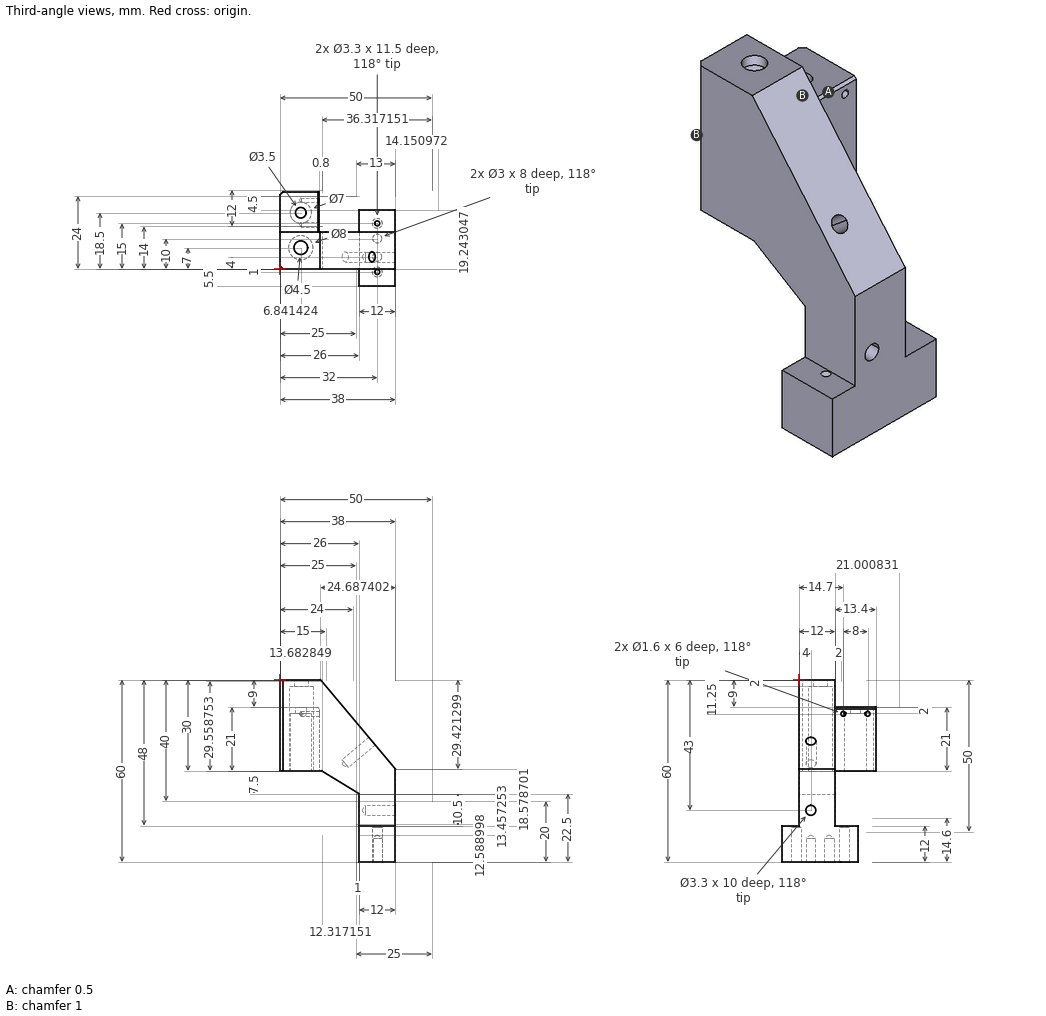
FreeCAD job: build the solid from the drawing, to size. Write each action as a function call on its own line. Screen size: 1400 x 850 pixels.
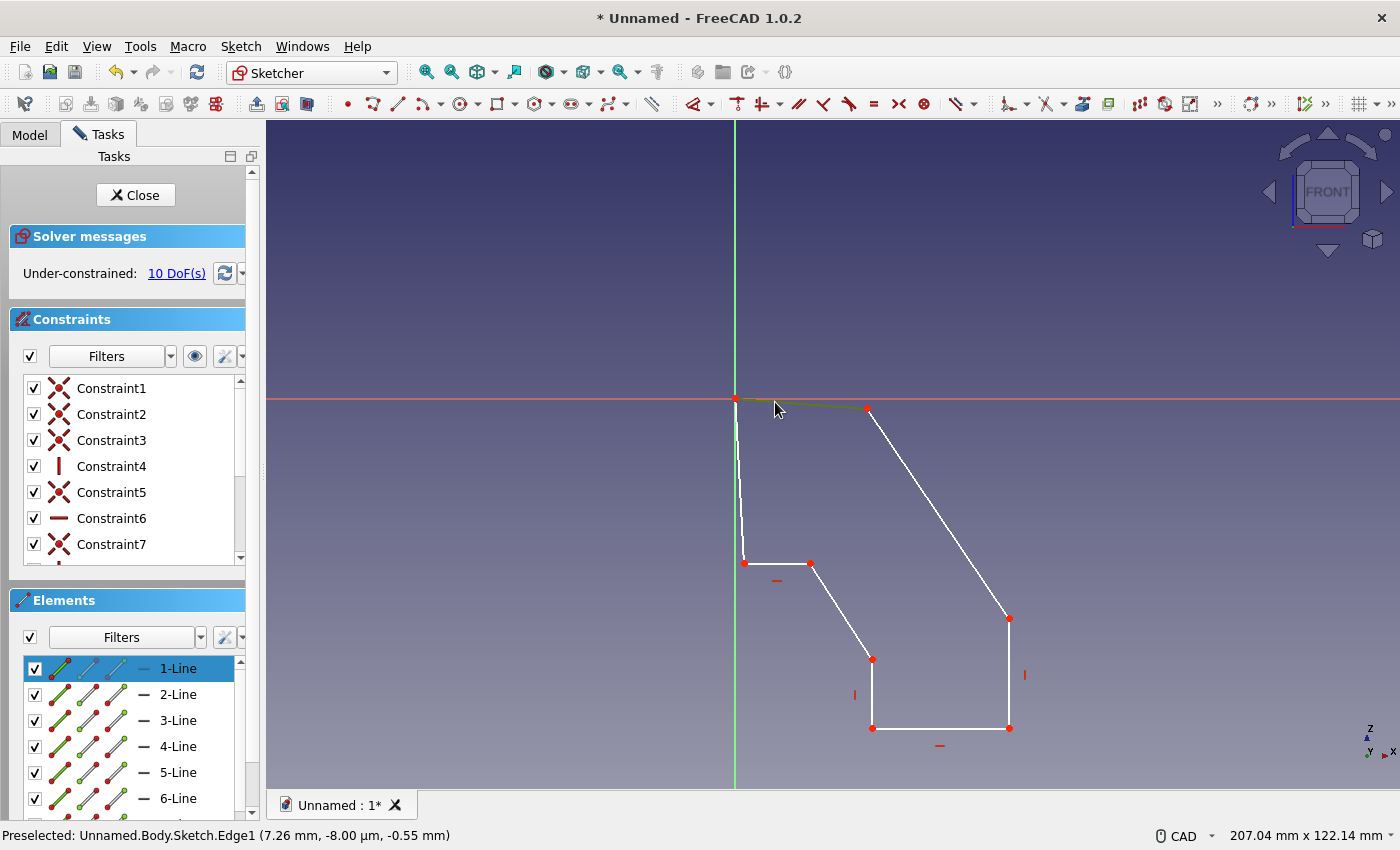
click(780, 104)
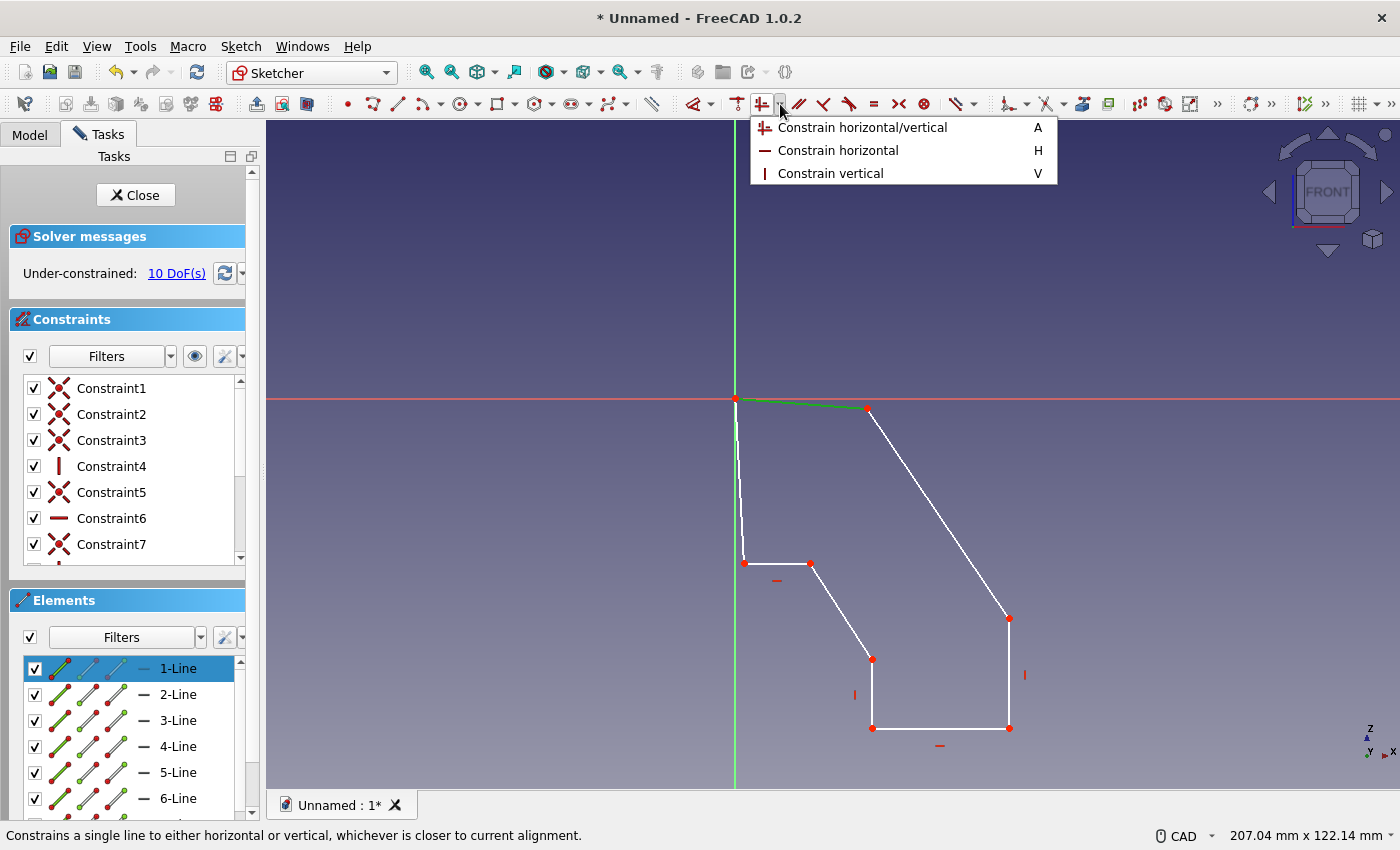
click(904, 150)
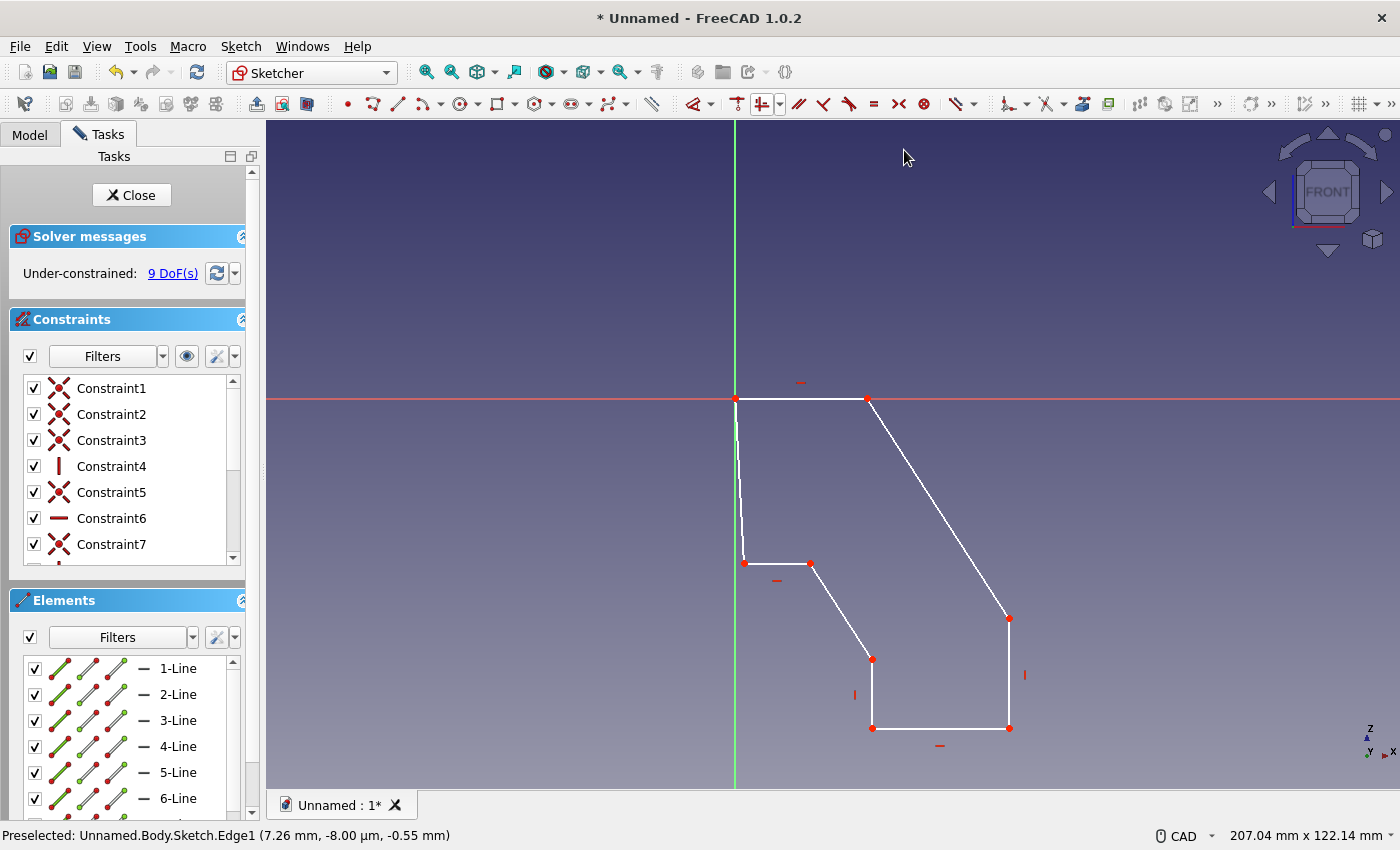
click(738, 448)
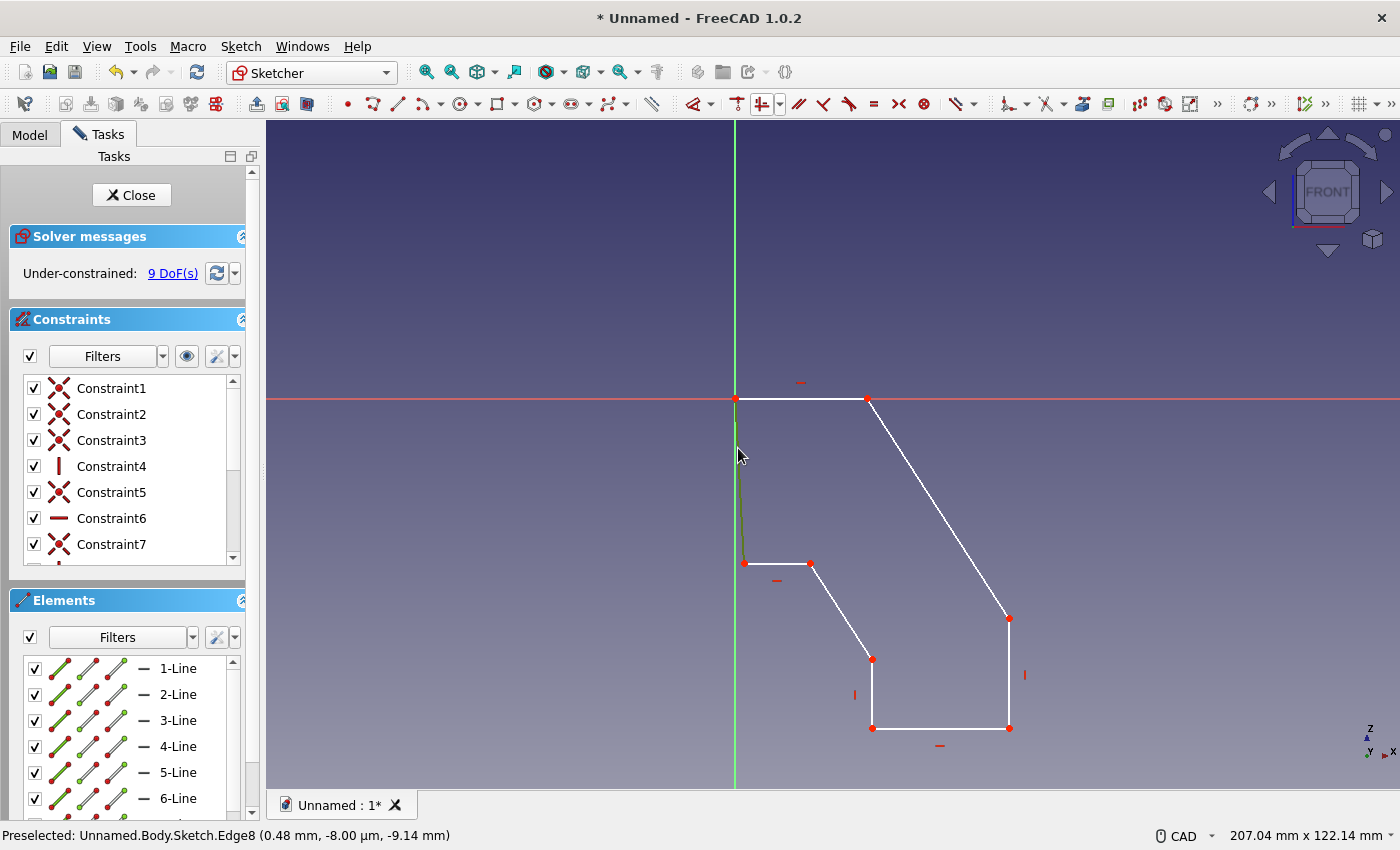
click(780, 104)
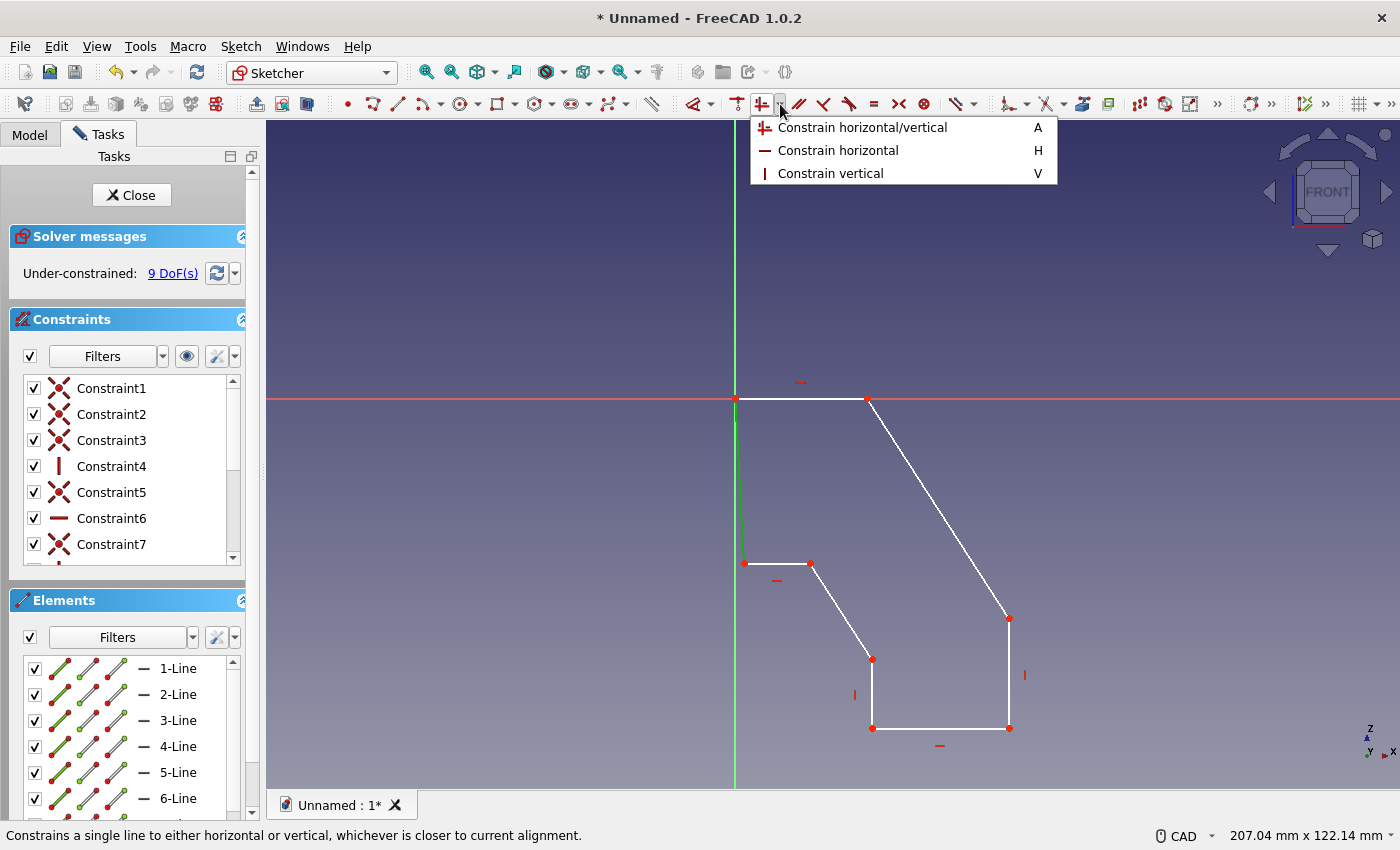
click(904, 174)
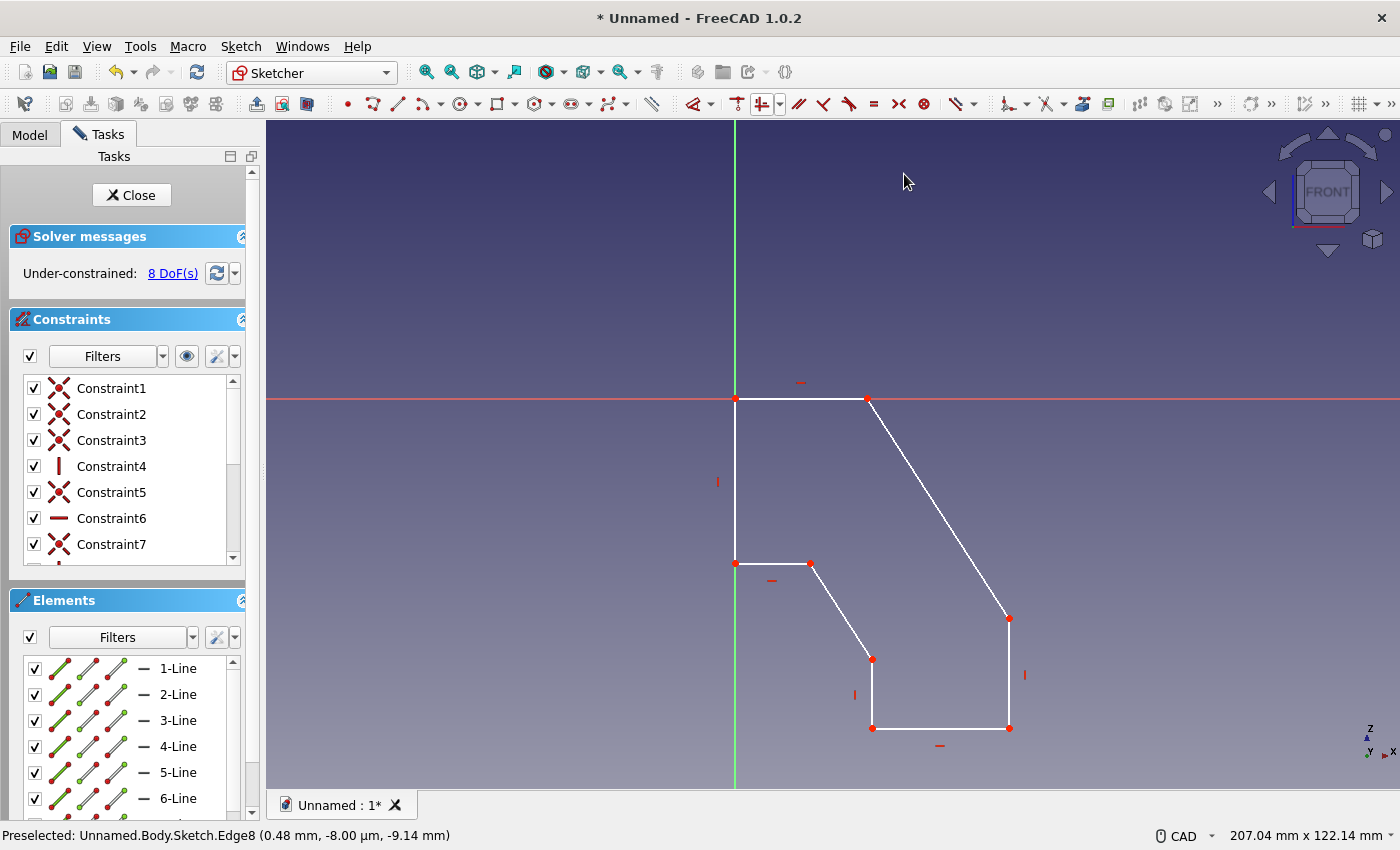
click(775, 399)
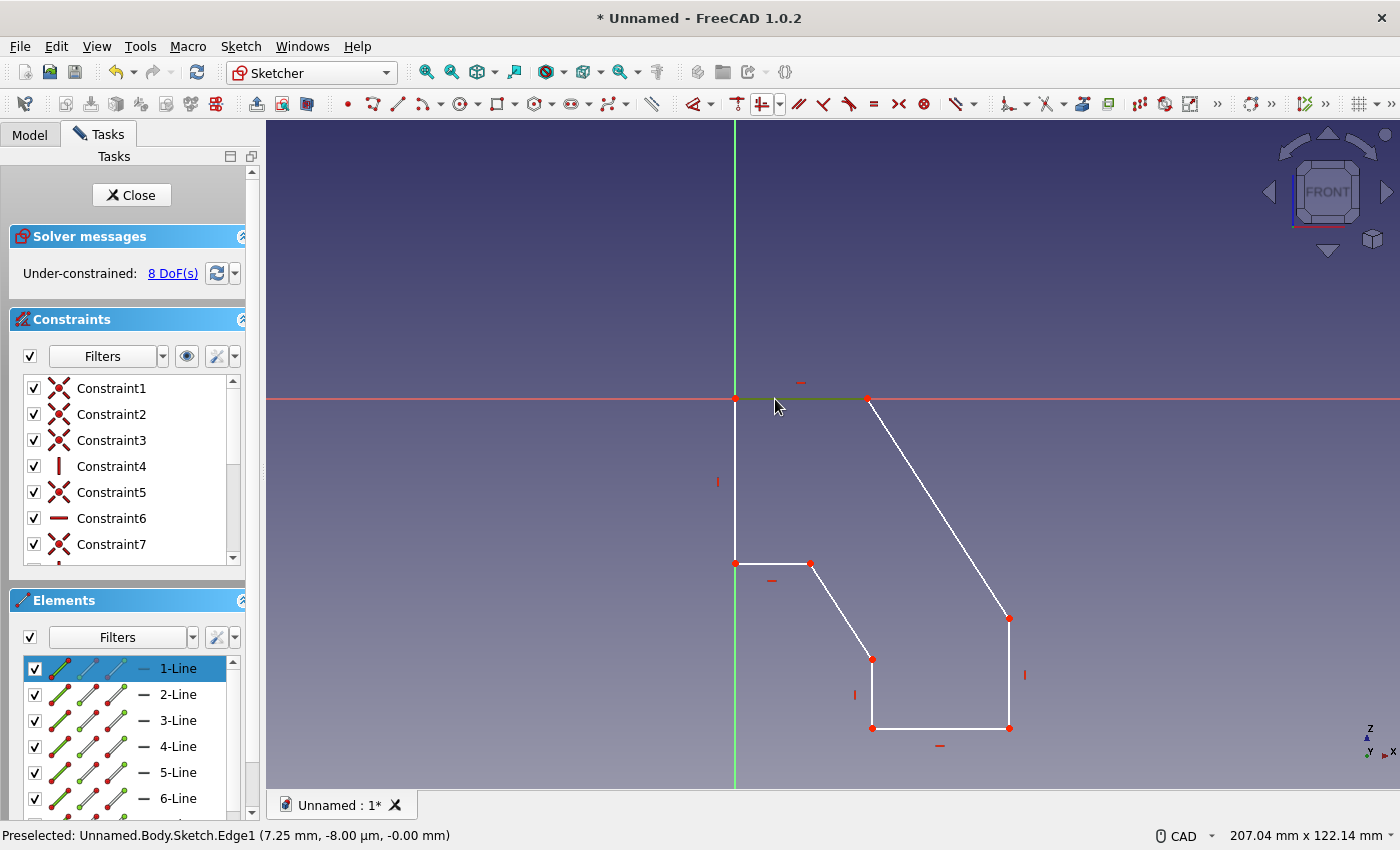
key(l)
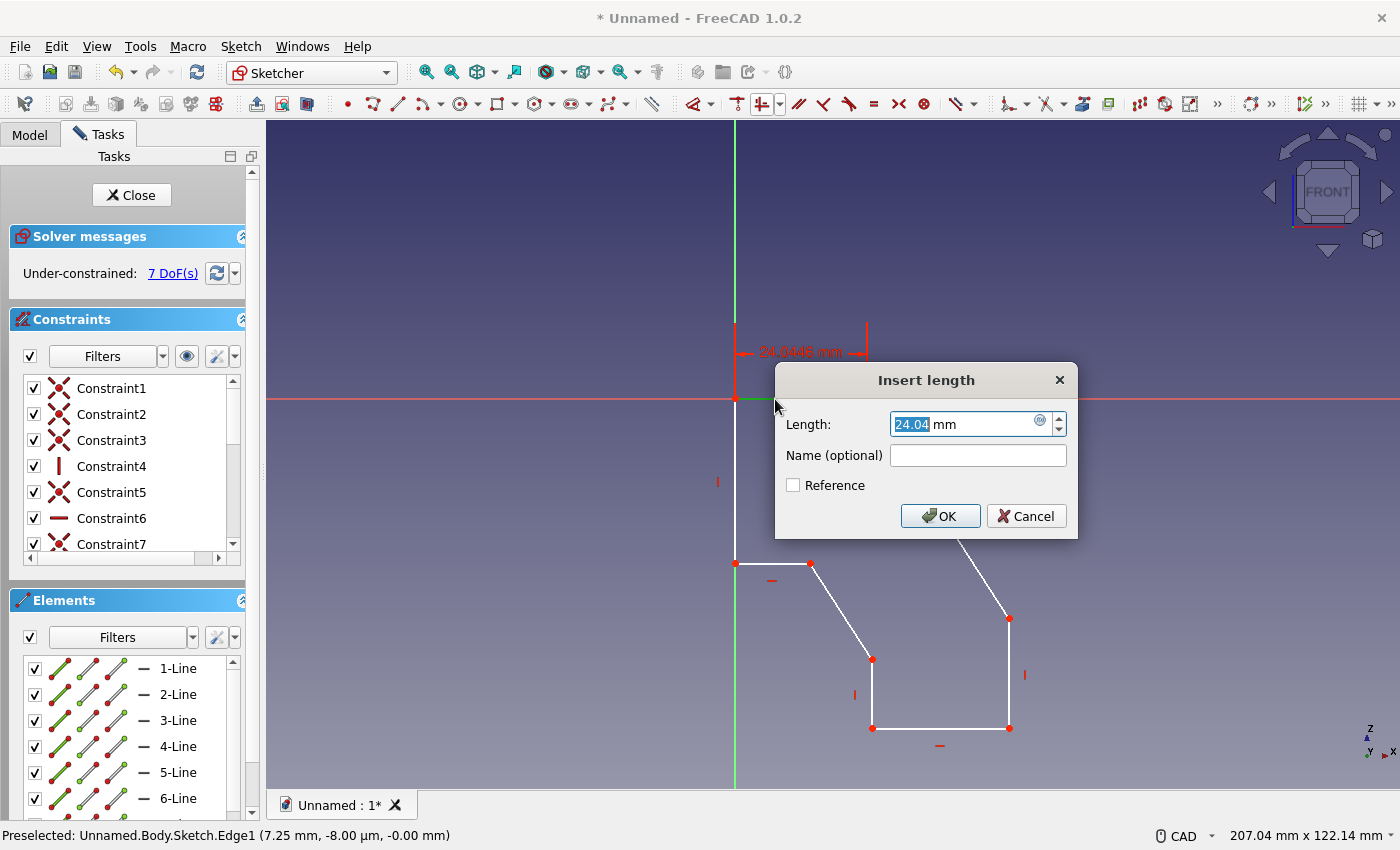
text(24)
key(Return)